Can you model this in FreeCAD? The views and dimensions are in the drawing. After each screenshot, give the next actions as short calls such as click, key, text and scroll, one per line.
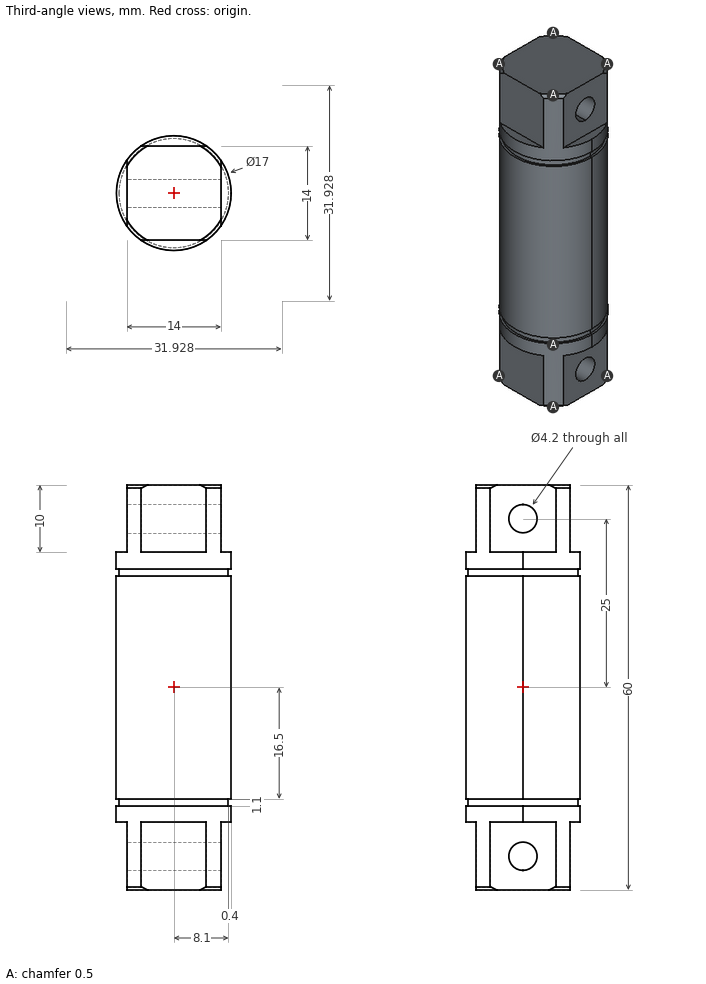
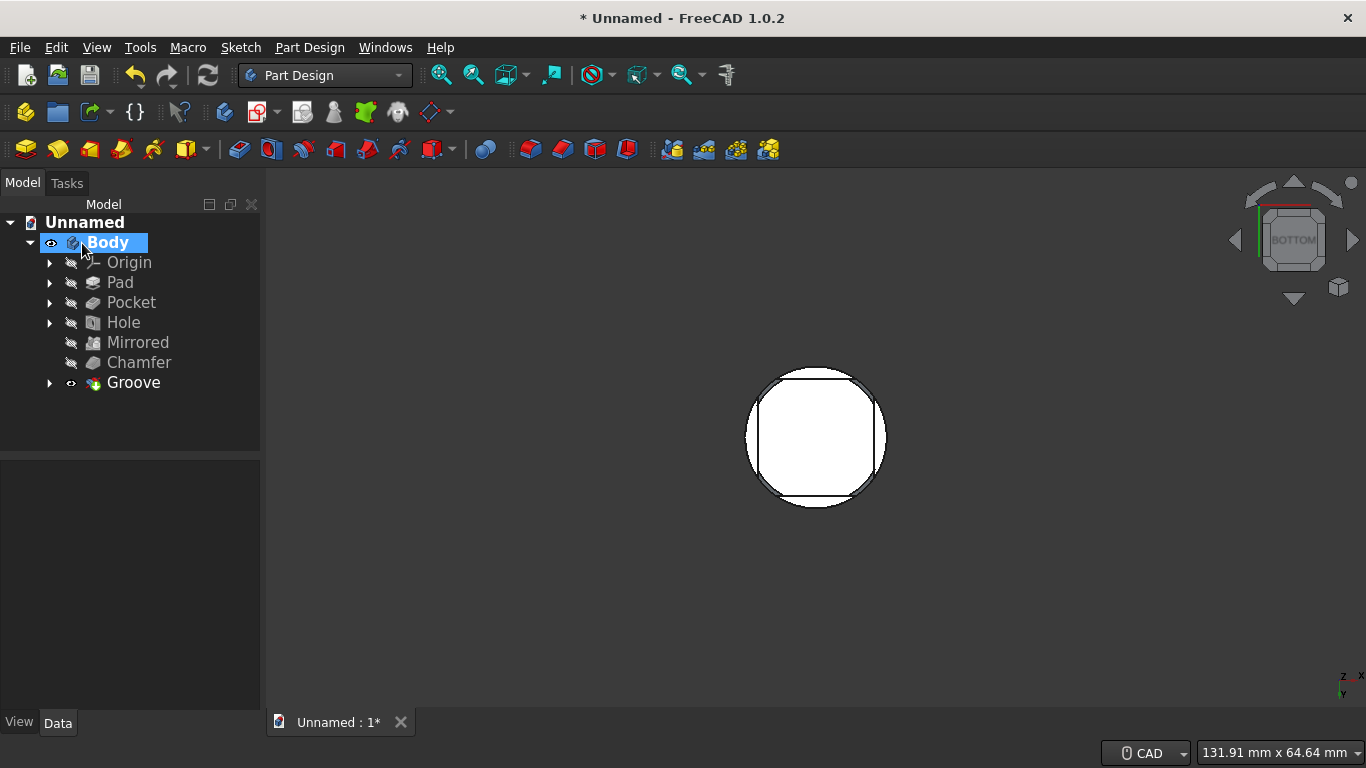
click(116, 383)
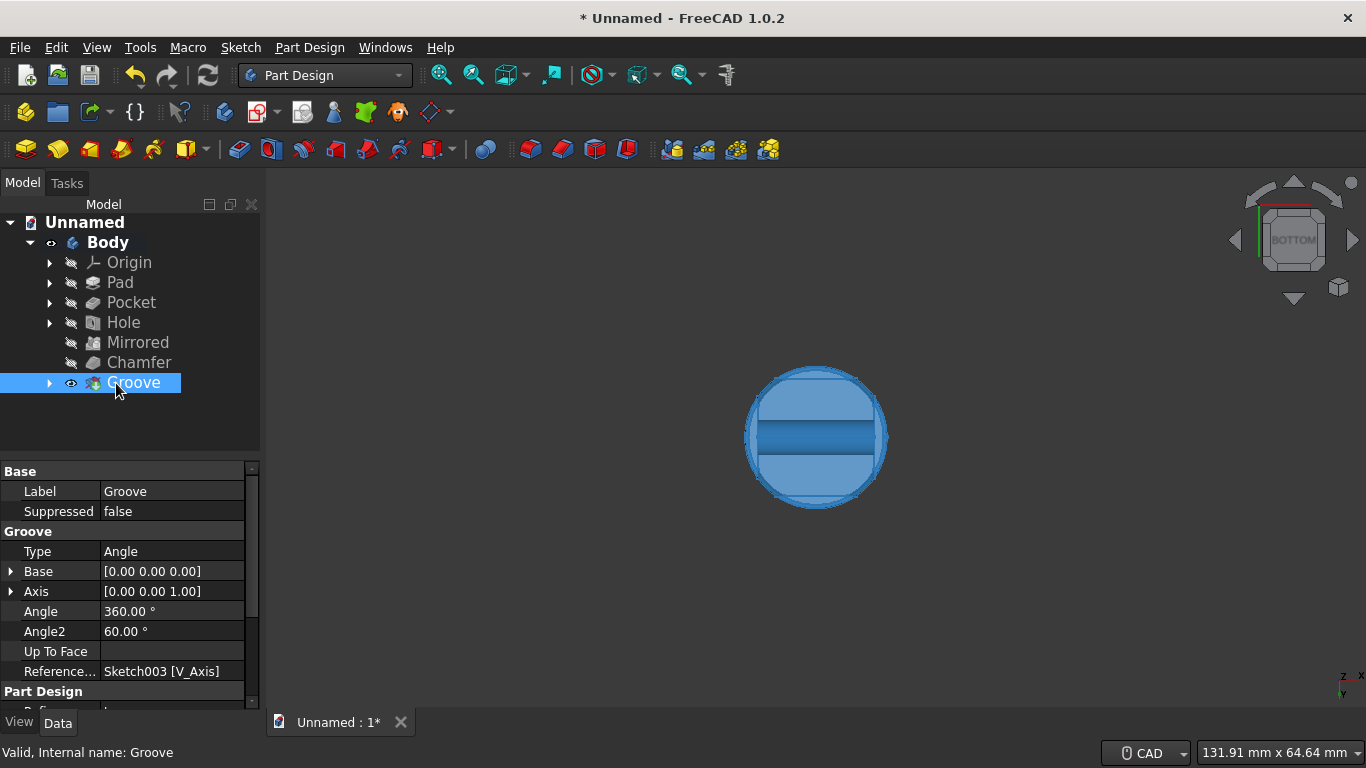
click(672, 150)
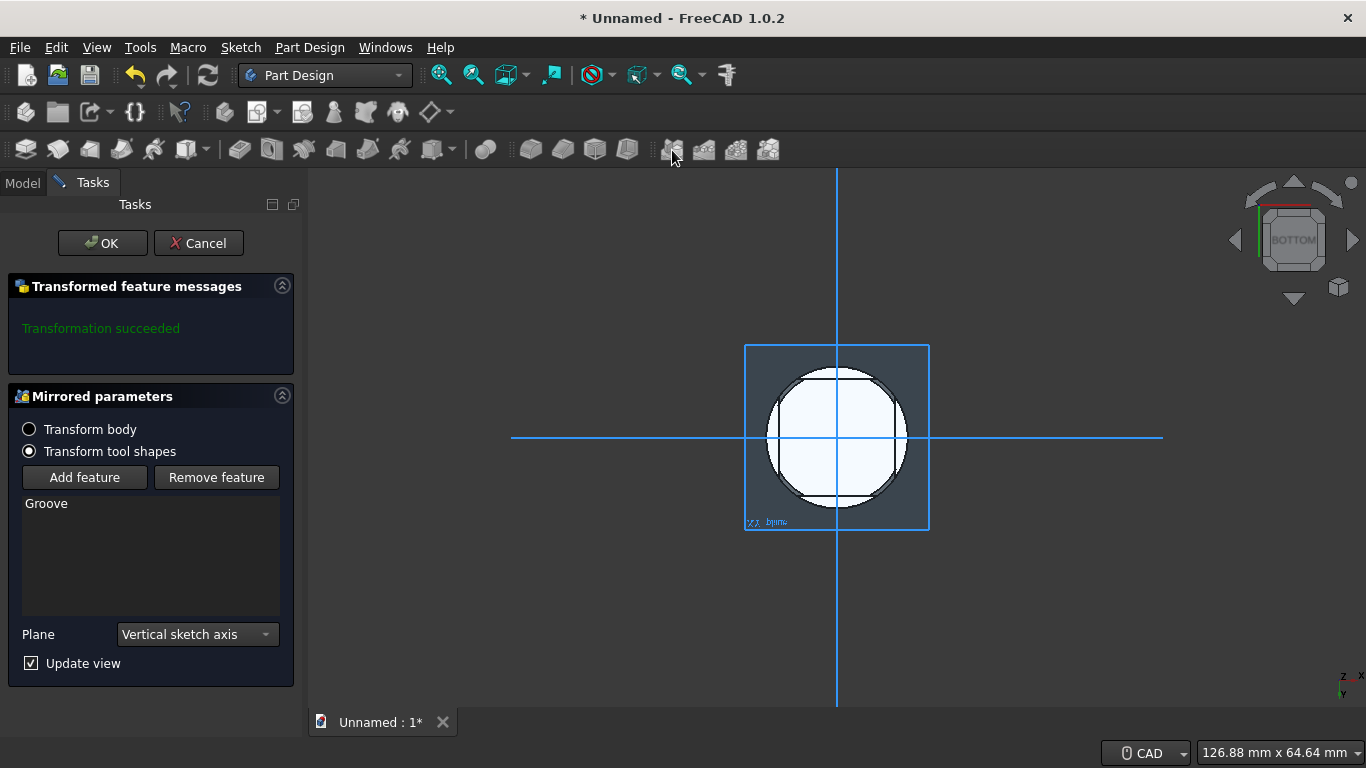
click(198, 634)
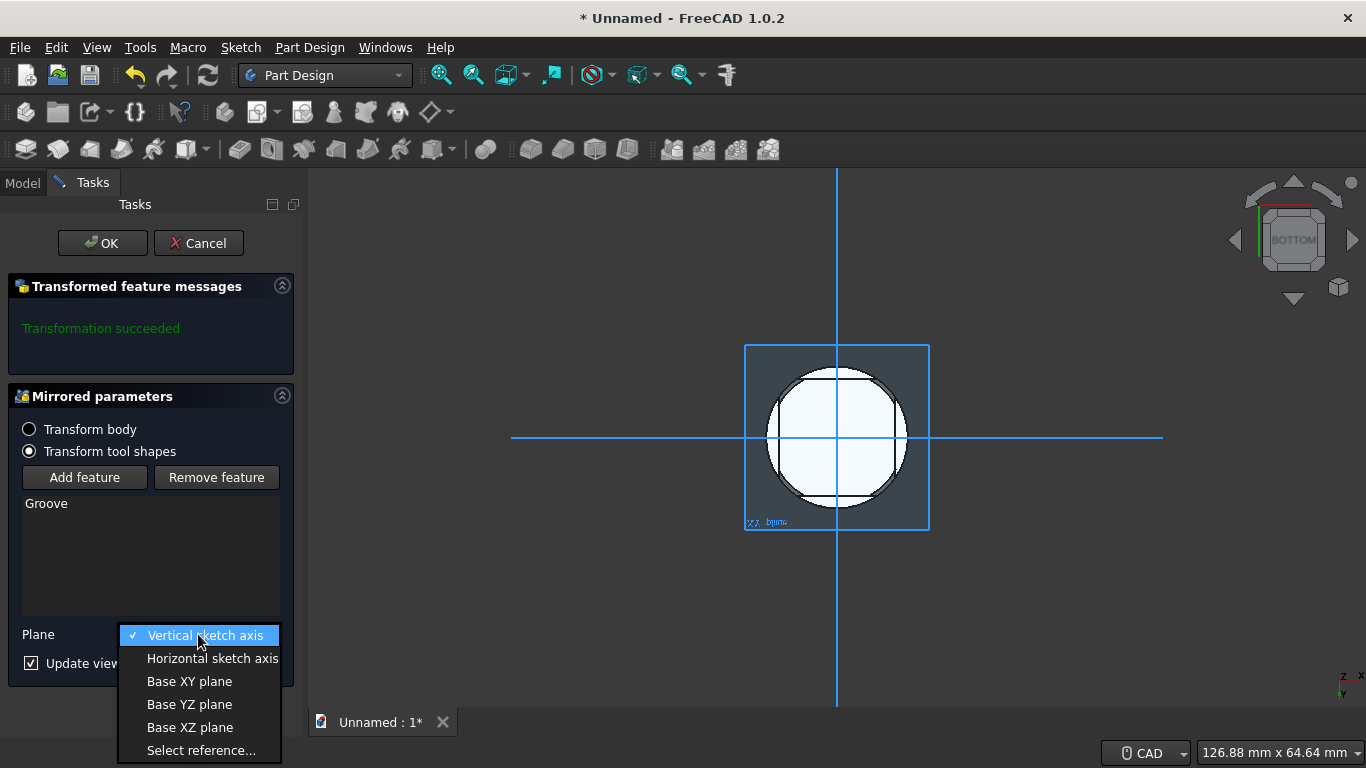
click(198, 682)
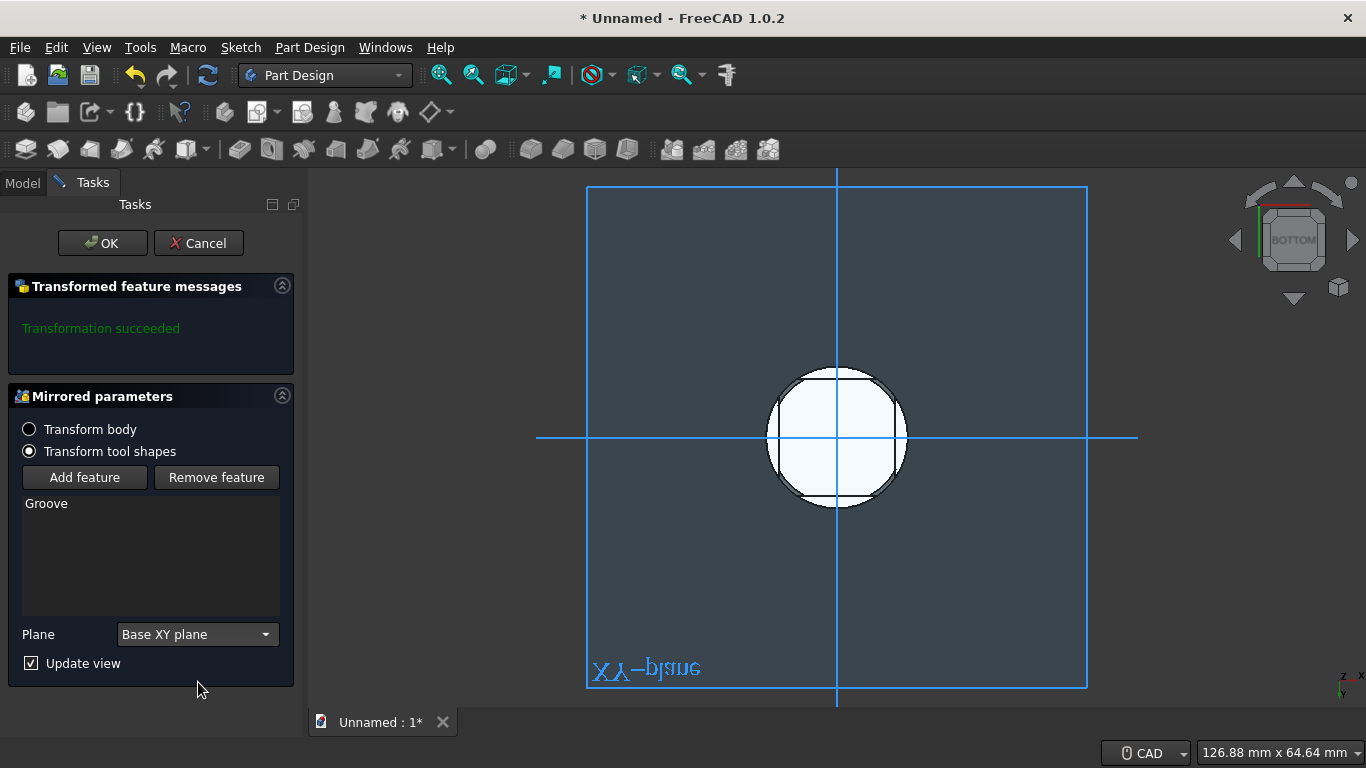
click(103, 243)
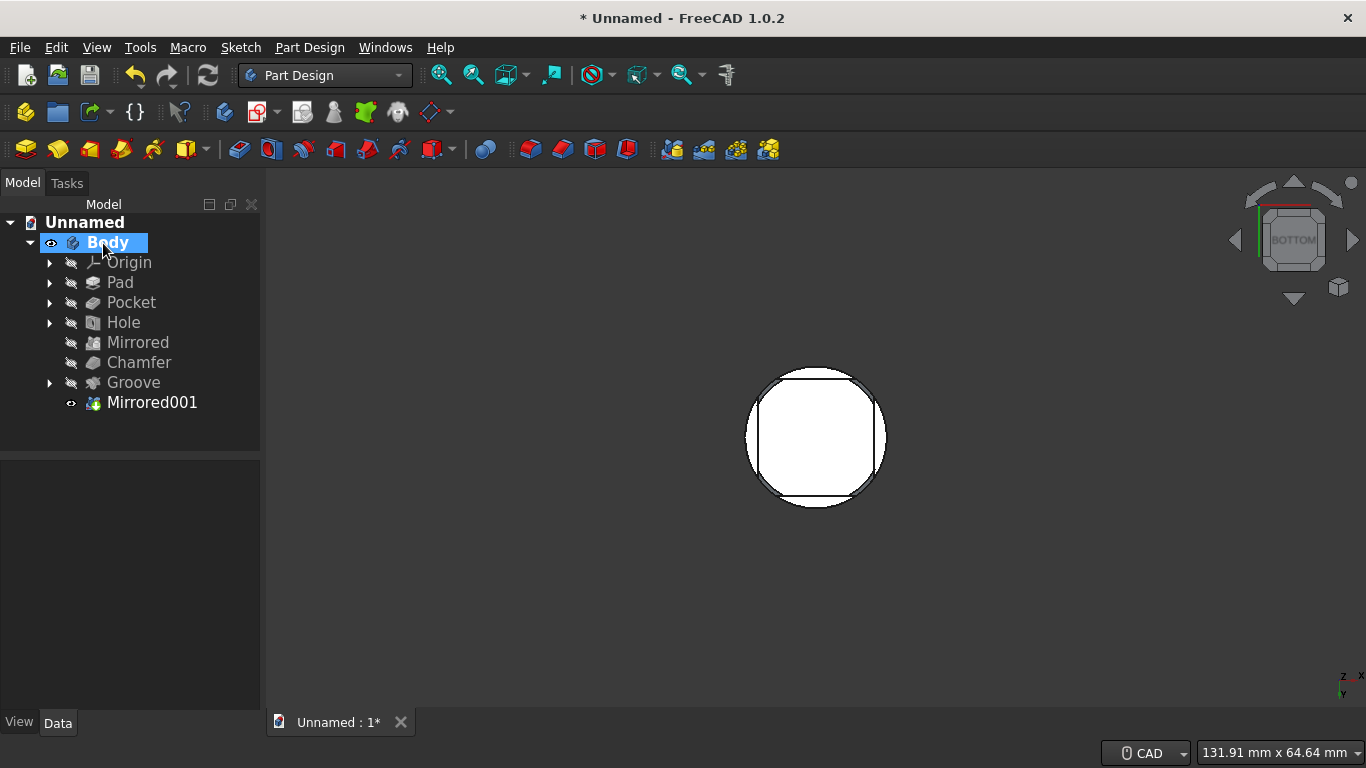
key(0)